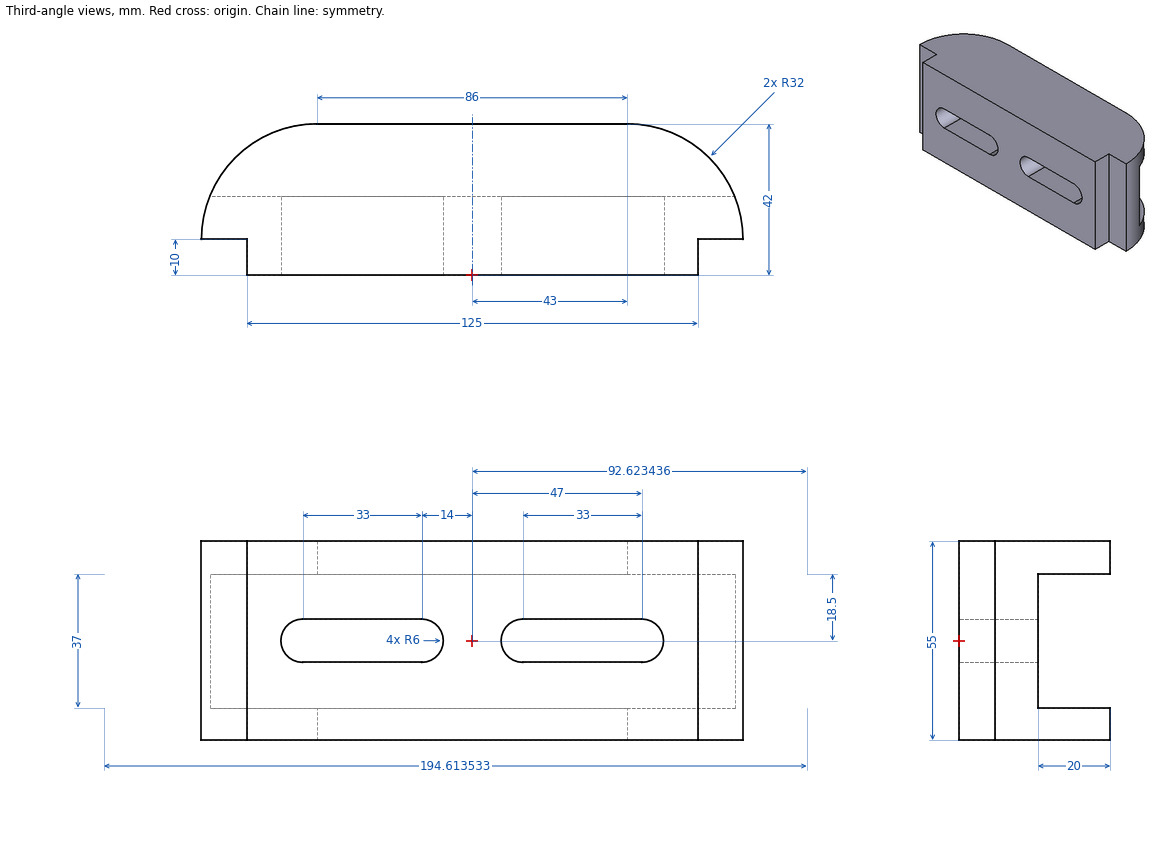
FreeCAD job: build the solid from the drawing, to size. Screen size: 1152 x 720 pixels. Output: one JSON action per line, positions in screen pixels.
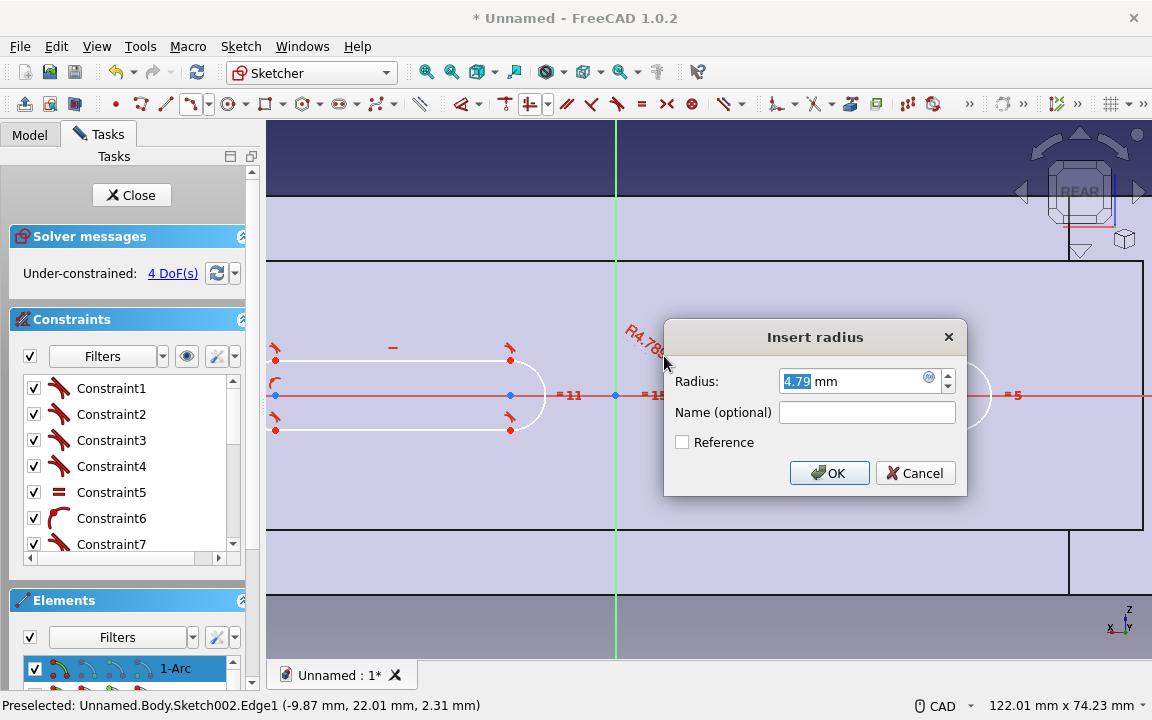
{"action": "type", "text": "6"}
{"action": "key", "text": "Return"}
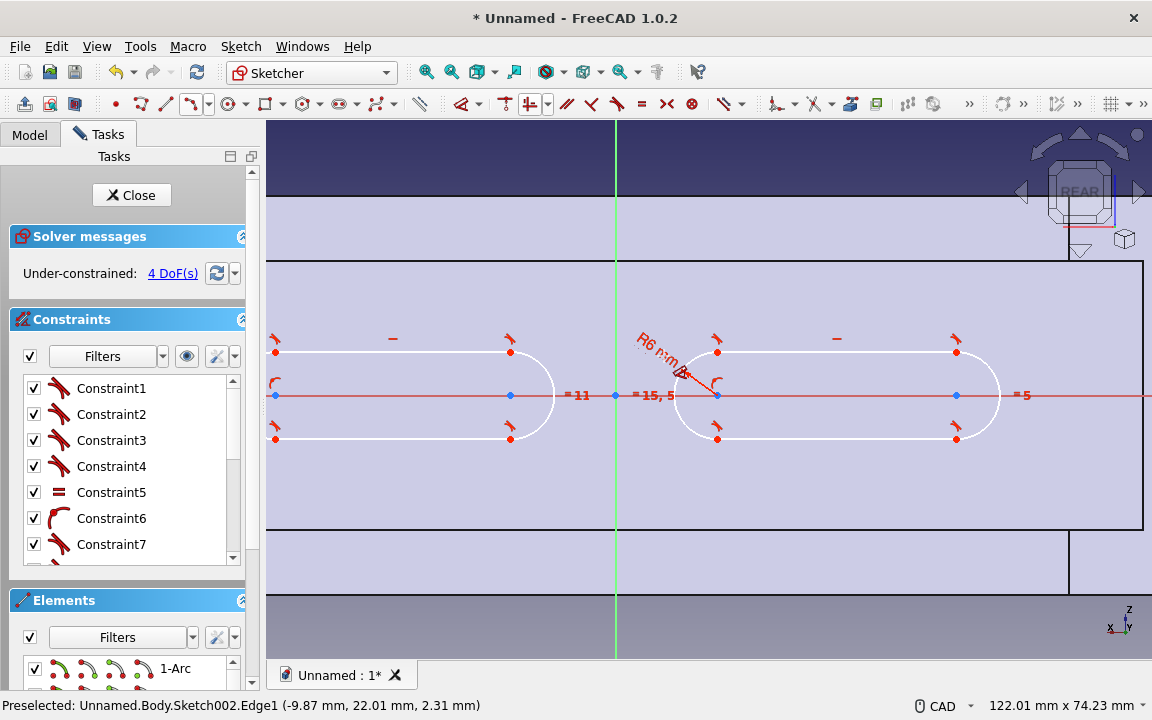
{"action": "left_click", "coordinate": [789, 352]}
{"action": "left_click", "coordinate": [837, 318]}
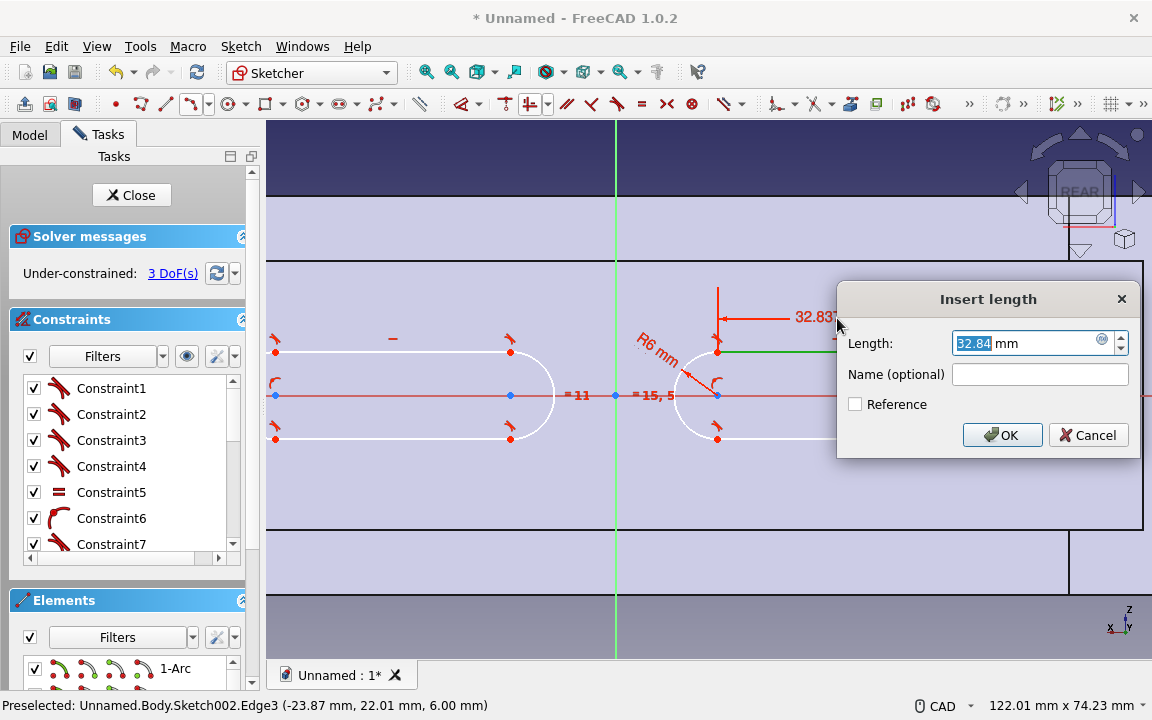
{"action": "type", "text": "33"}
{"action": "key", "text": "Return"}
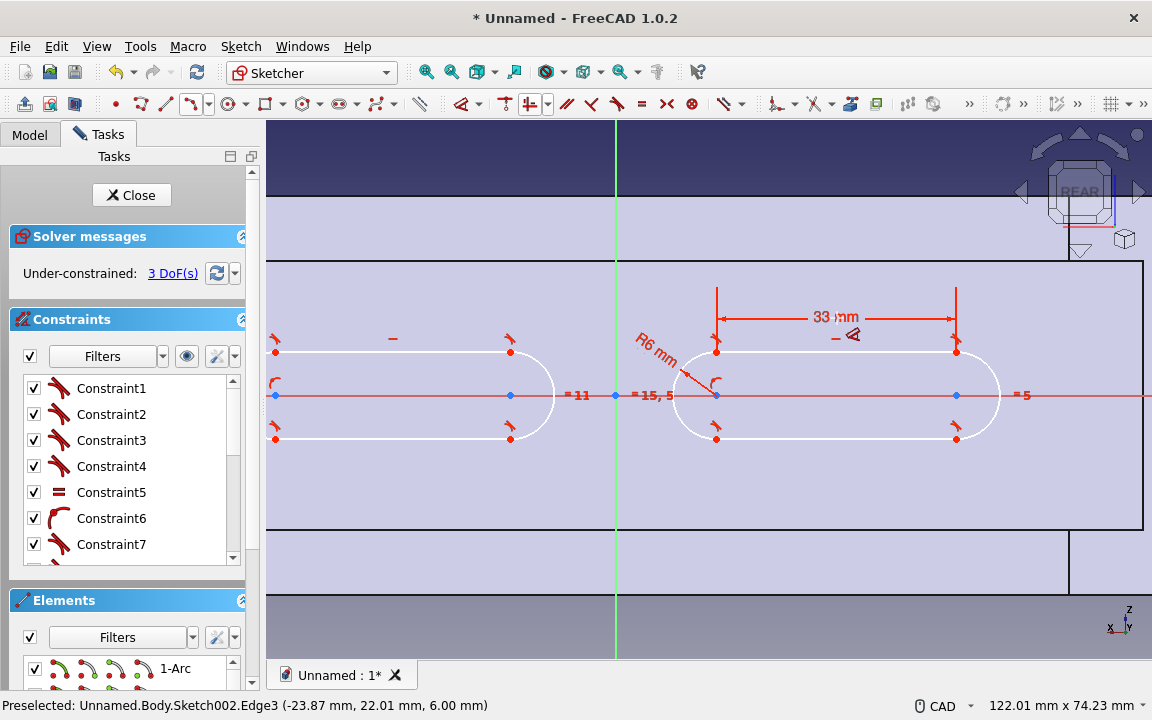
{"action": "left_click", "coordinate": [346, 352]}
{"action": "left_click", "coordinate": [402, 318]}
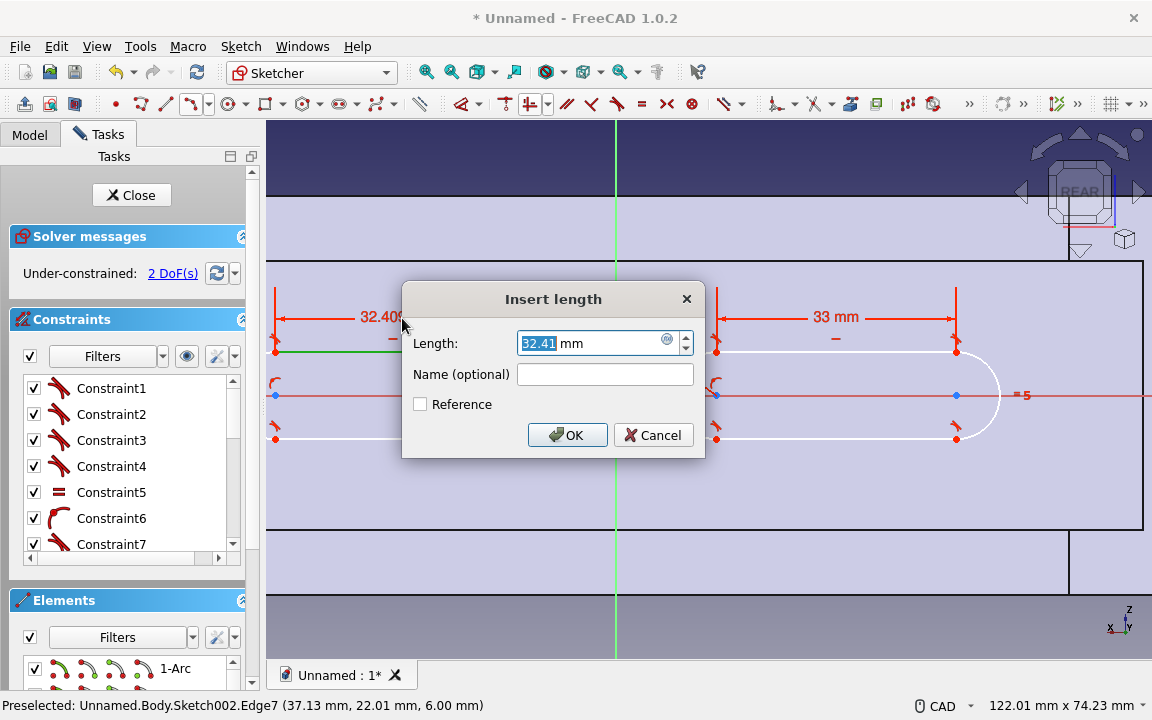
{"action": "type", "text": "33"}
{"action": "key", "text": "Return"}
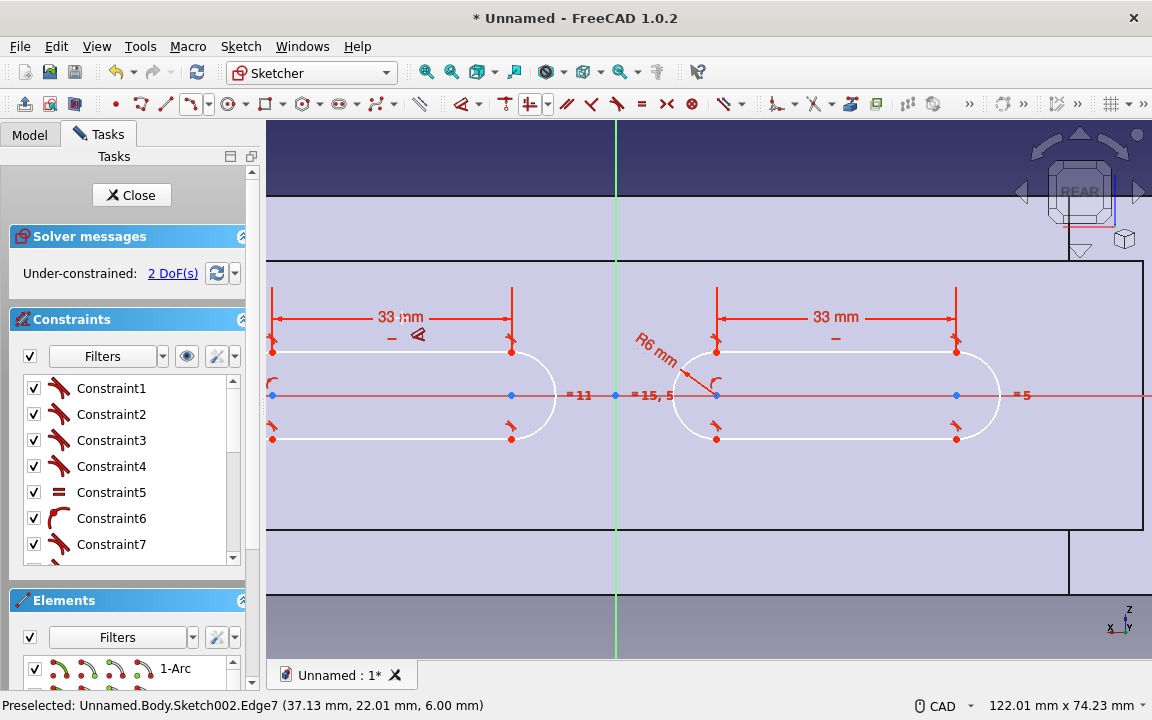
{"action": "left_click", "coordinate": [717, 352]}
{"action": "left_click", "coordinate": [666, 318]}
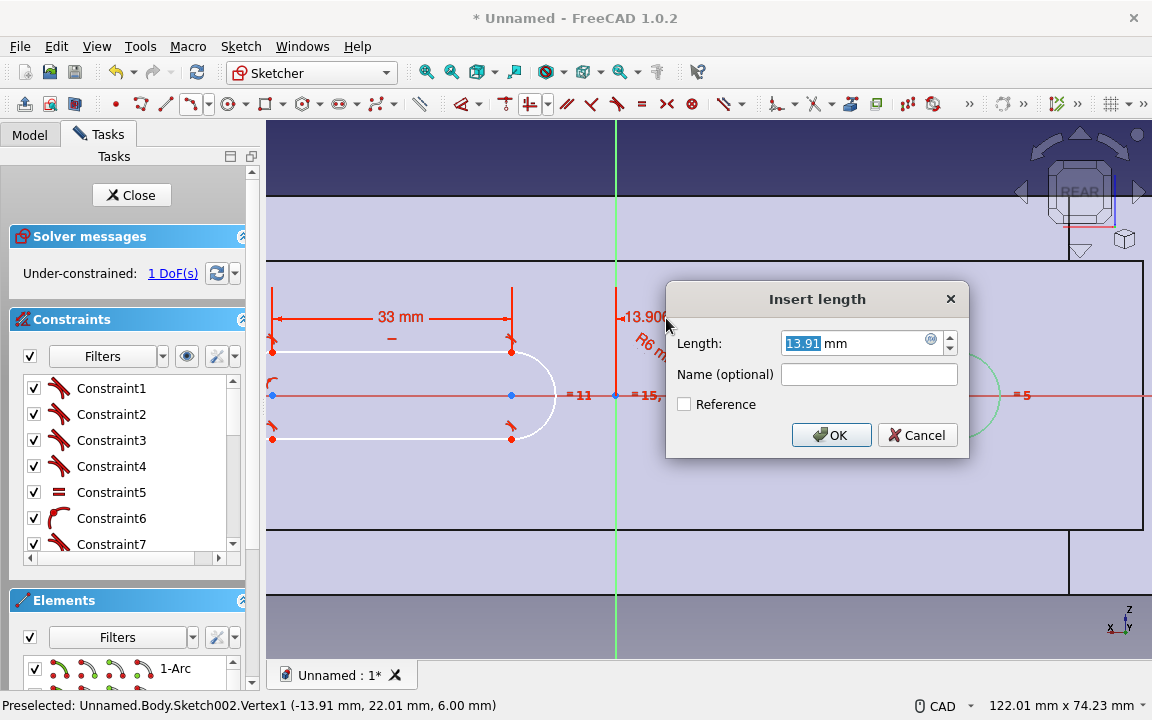
{"action": "type", "text": "14"}
{"action": "key", "text": "Return"}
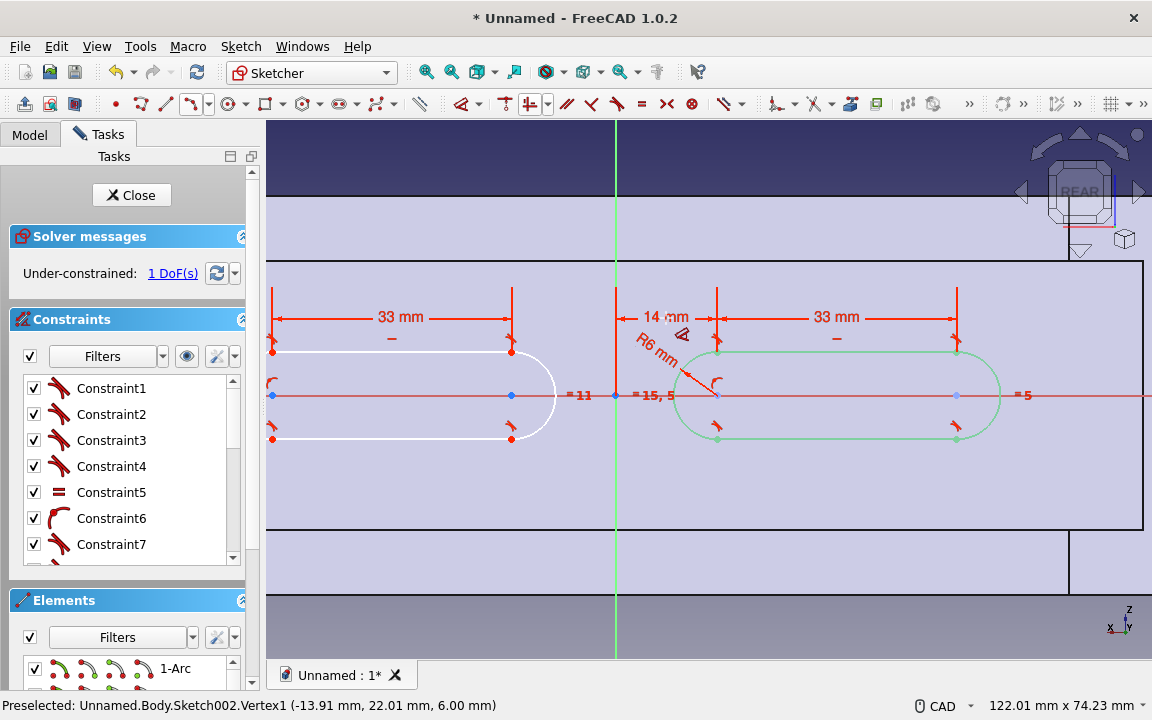
{"action": "scroll", "coordinate": [691, 377], "scroll_direction": "down", "scroll_amount": 2}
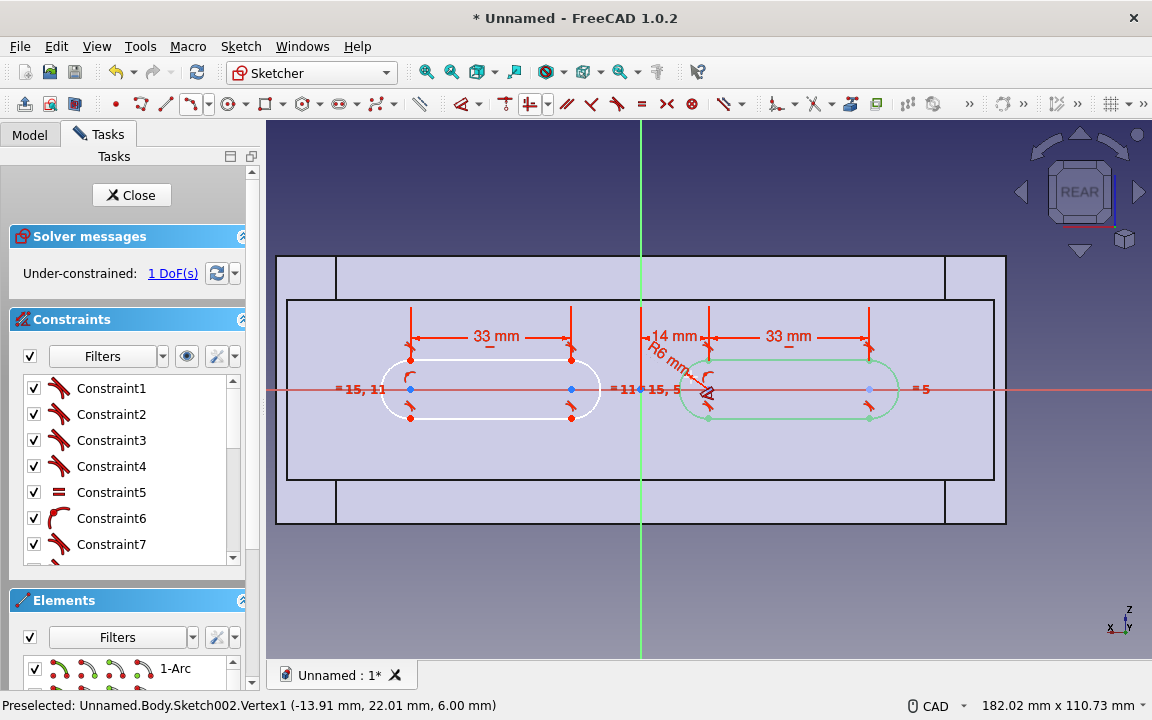
{"action": "left_click", "coordinate": [411, 360]}
{"action": "left_click", "coordinate": [579, 326]}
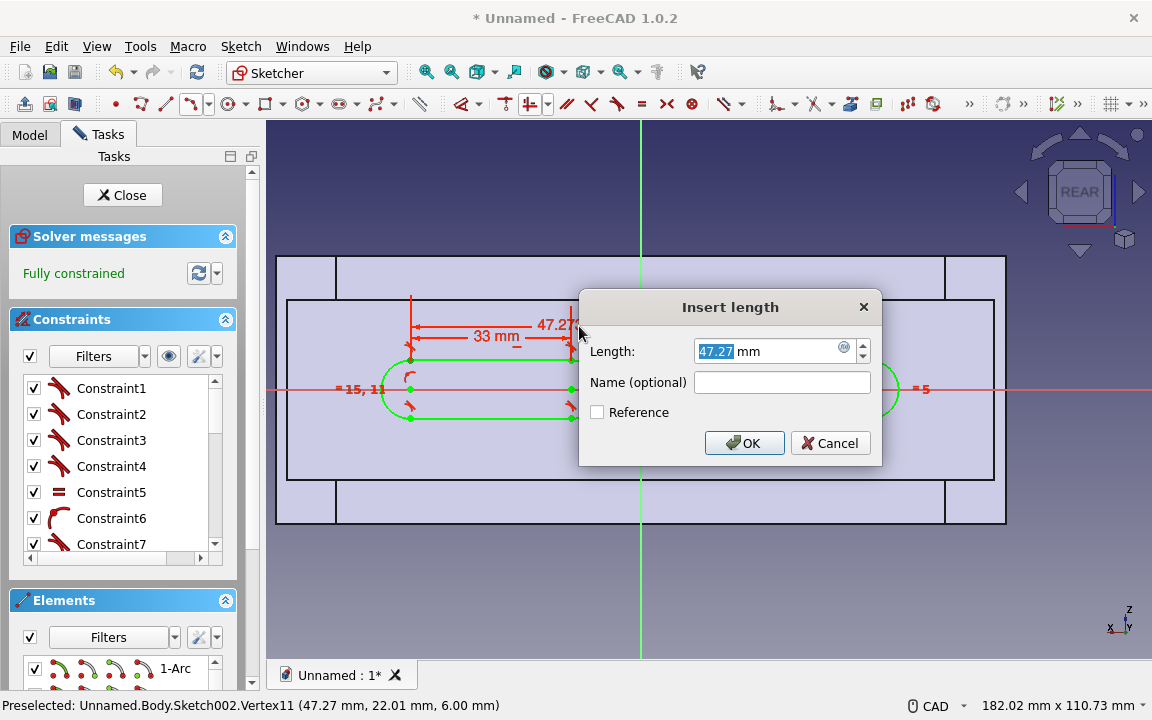
{"action": "type", "text": "47"}
{"action": "key", "text": "Return"}
{"action": "key", "text": "Escape"}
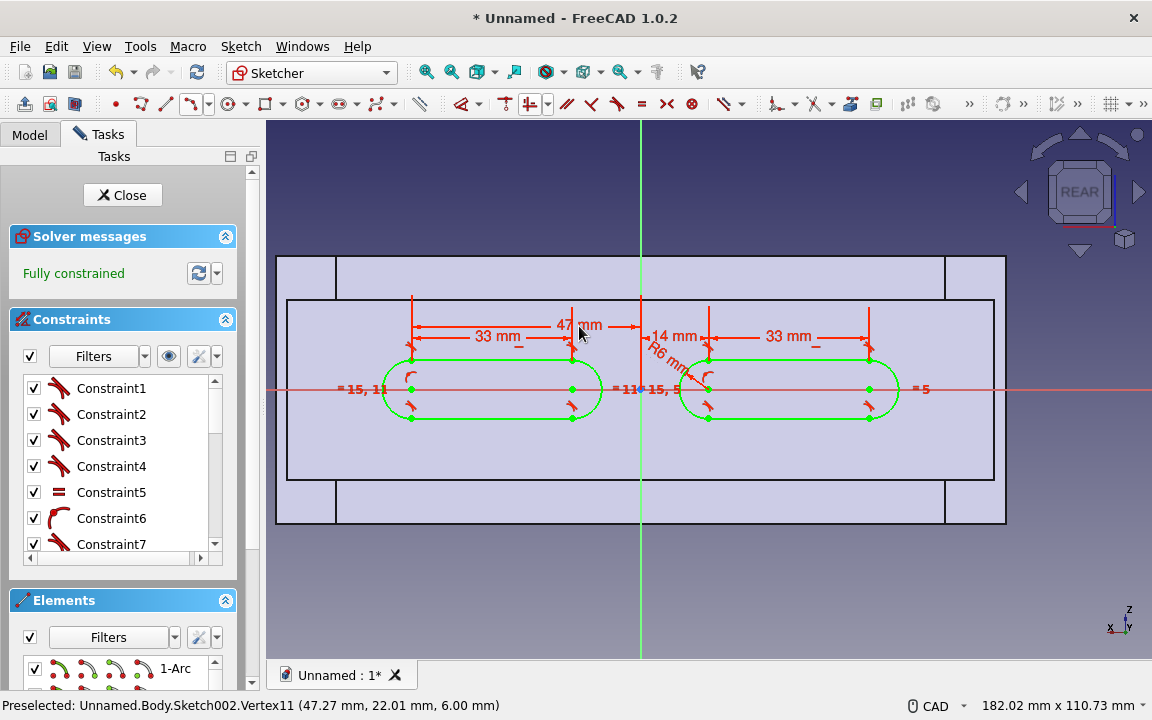
{"action": "left_click", "coordinate": [123, 195]}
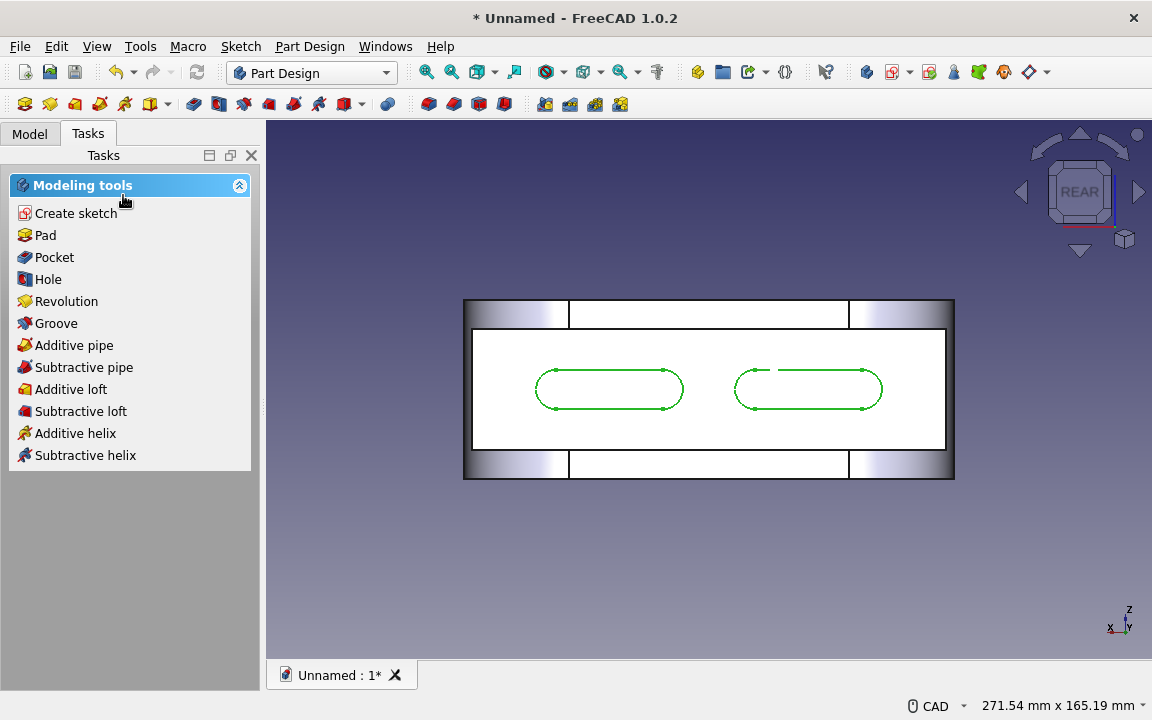
{"action": "left_click", "coordinate": [194, 104]}